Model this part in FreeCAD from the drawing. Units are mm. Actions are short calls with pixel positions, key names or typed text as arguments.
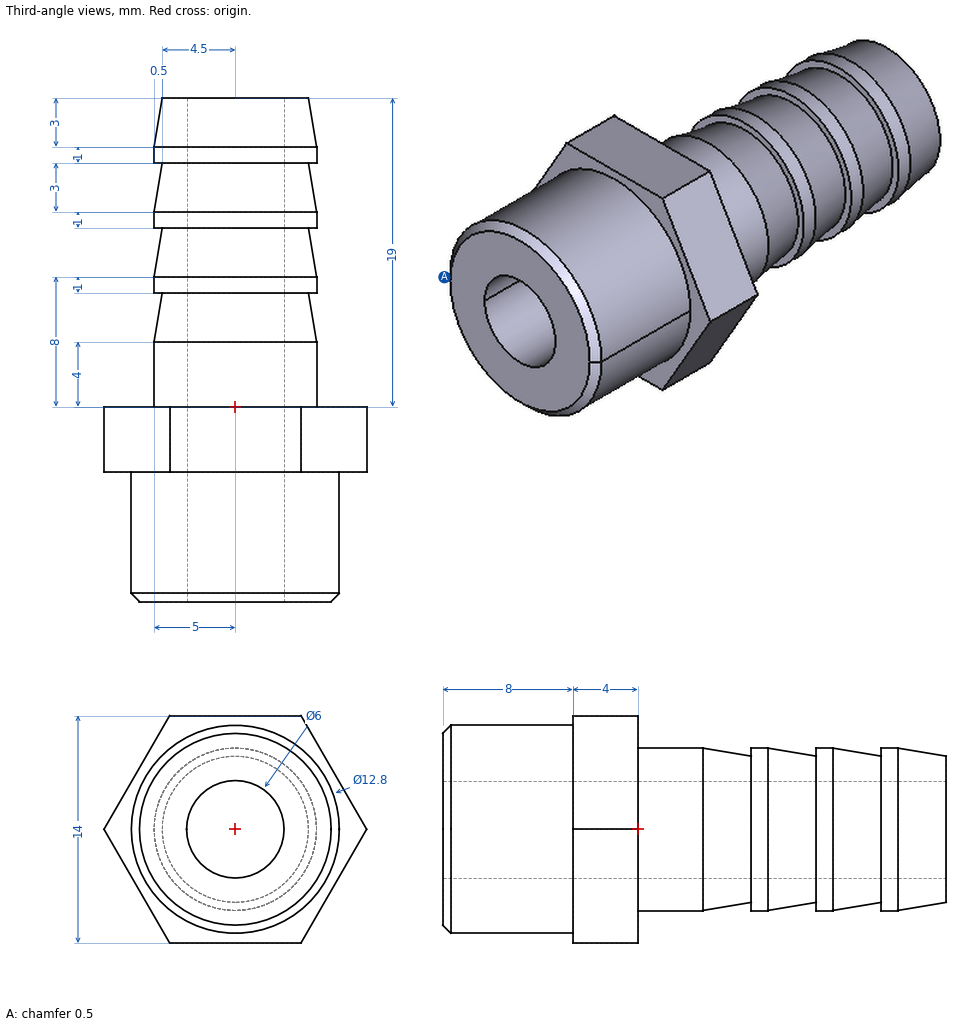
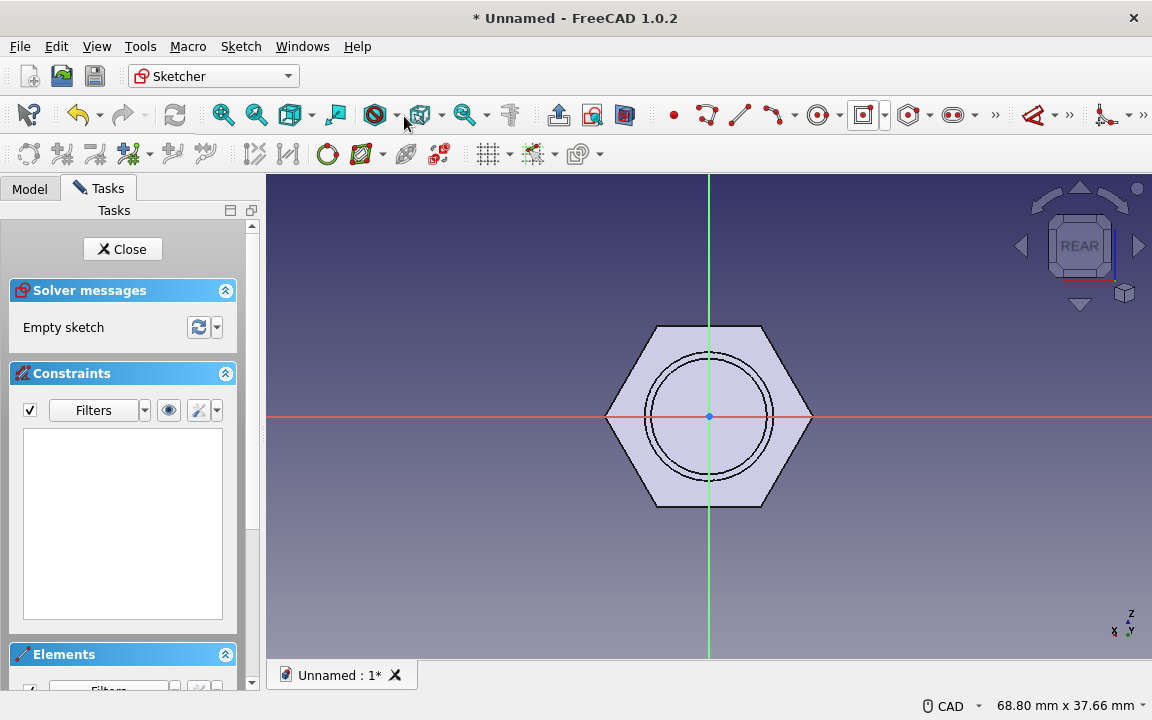
scroll(731, 417, up, 7)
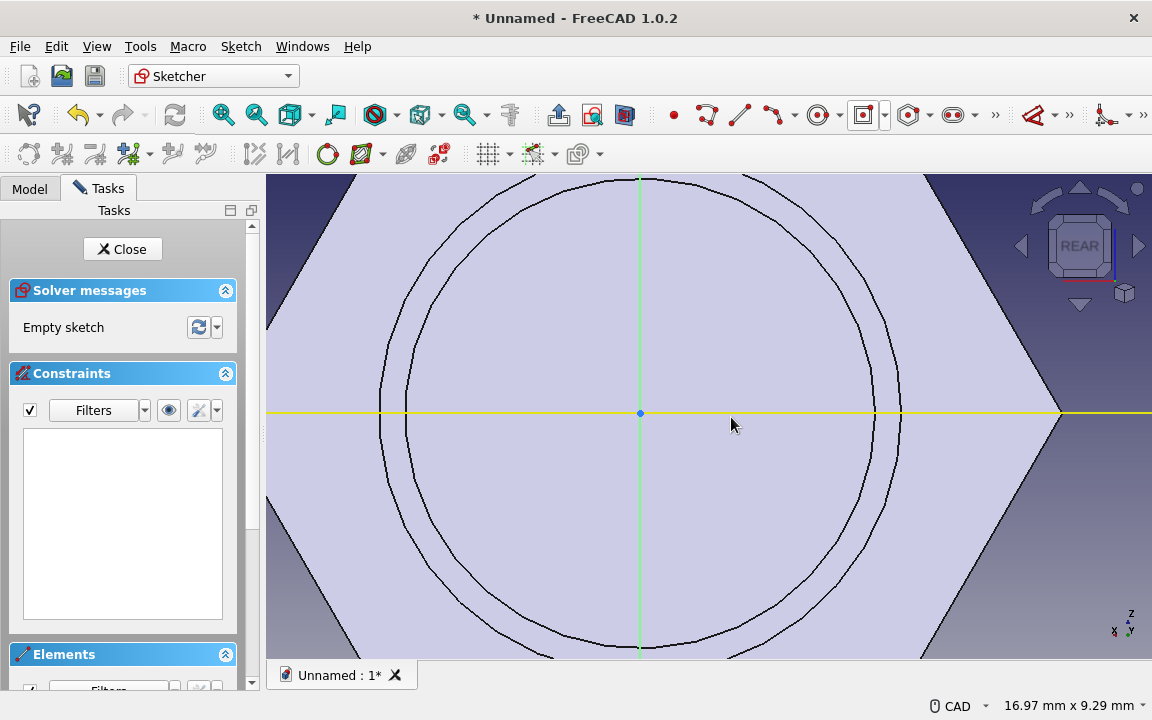
click(818, 116)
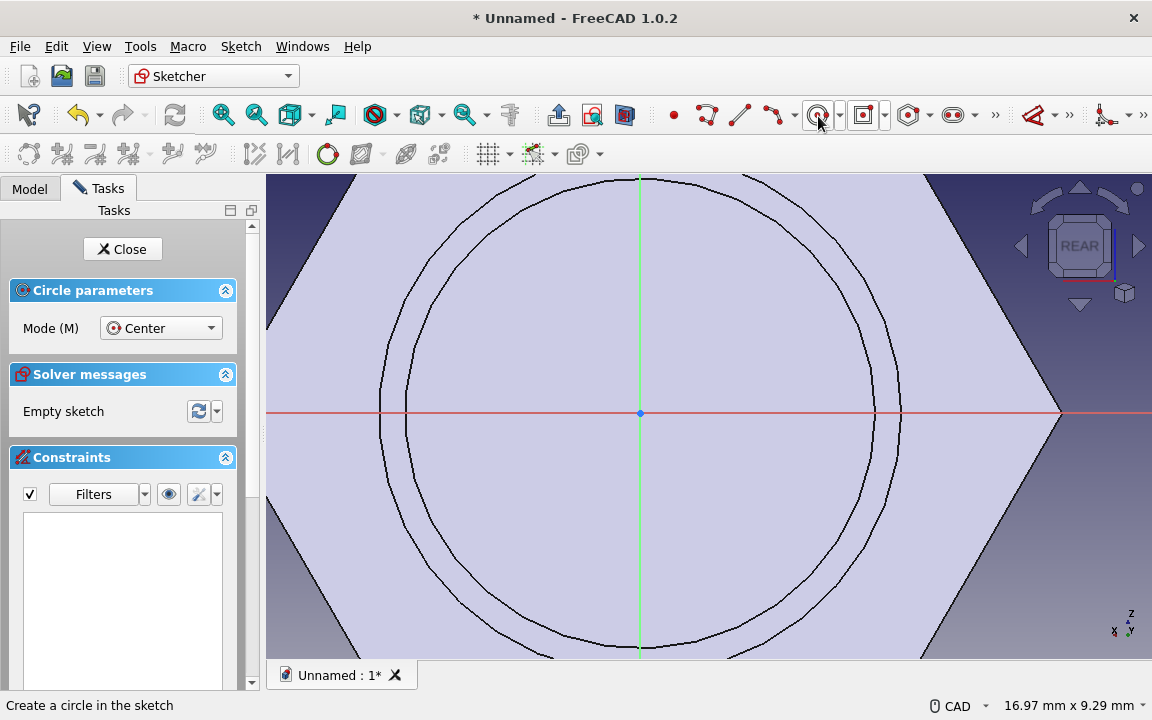
click(640, 413)
click(751, 303)
key(Escape)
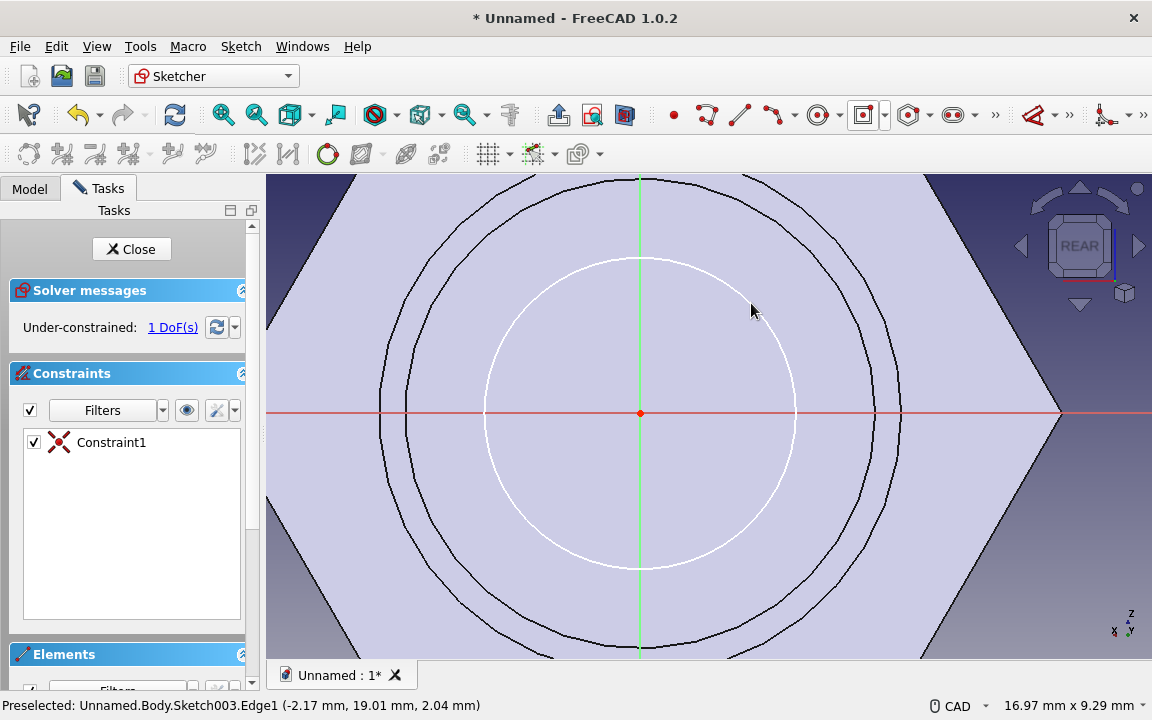
click(1032, 116)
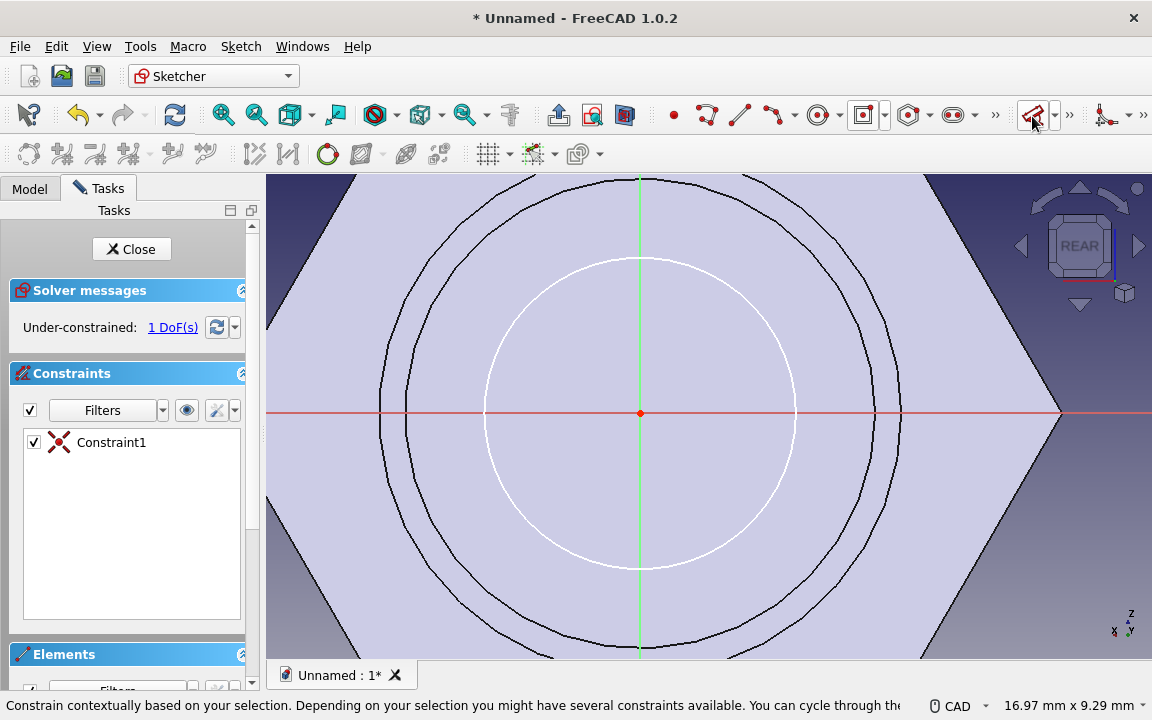
click(750, 303)
click(773, 280)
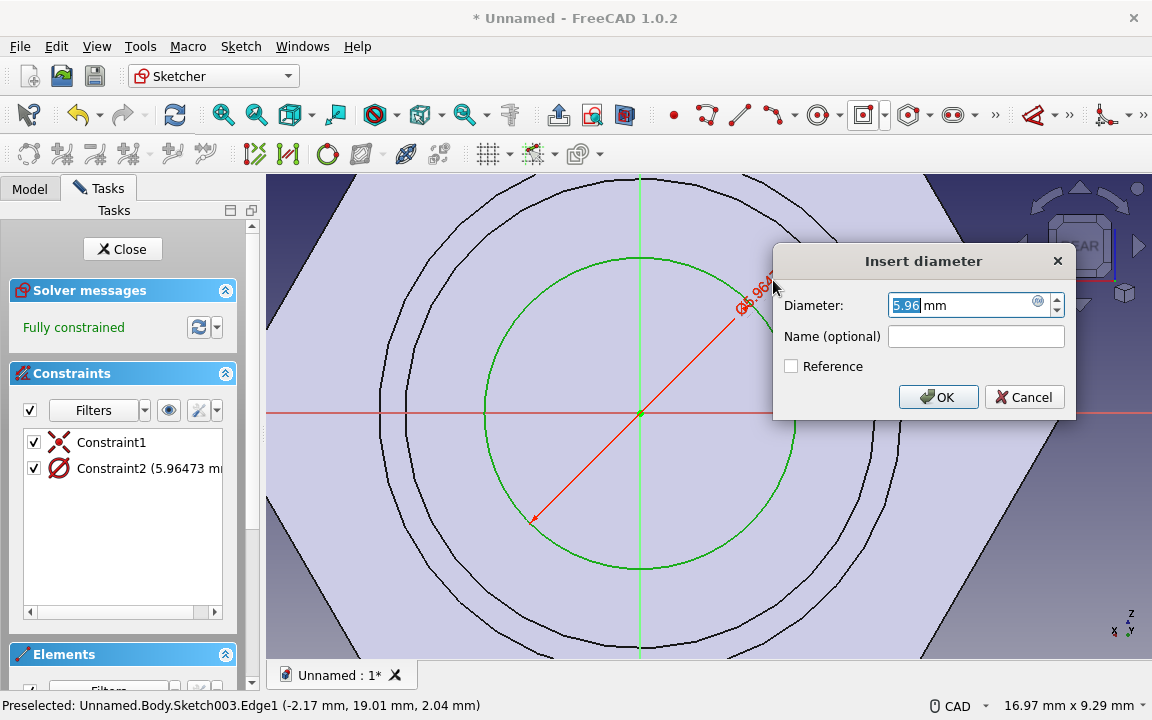
text(6)
key(Return)
key(Escape)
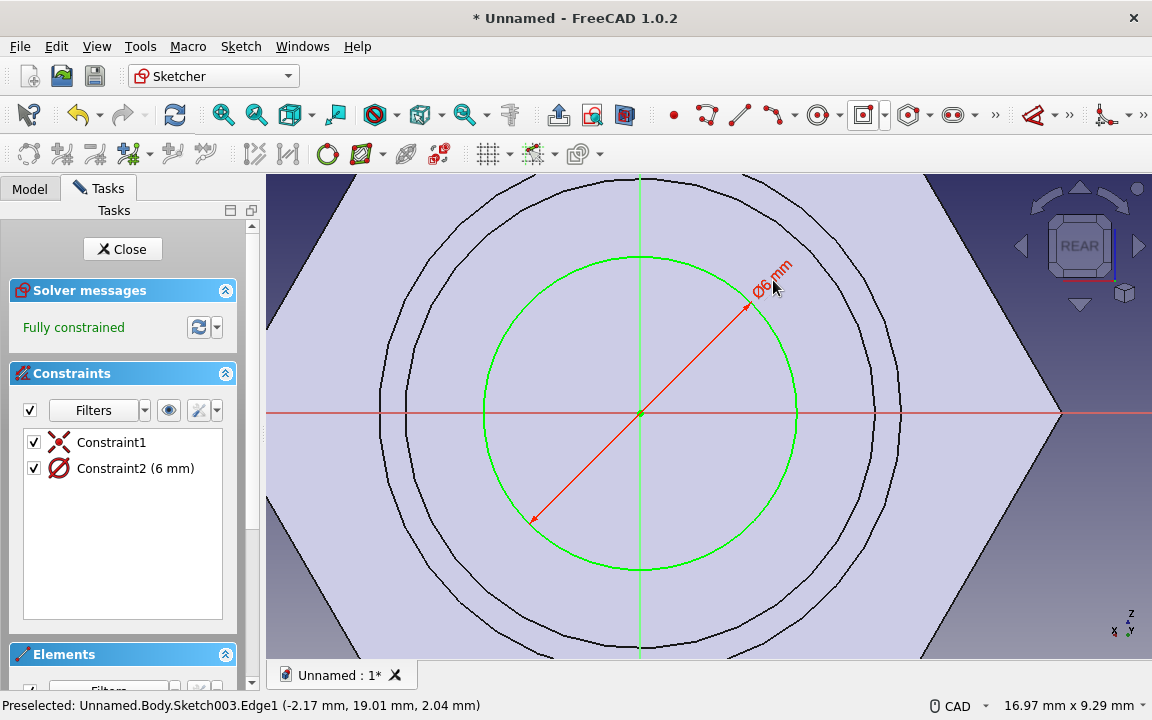
click(123, 249)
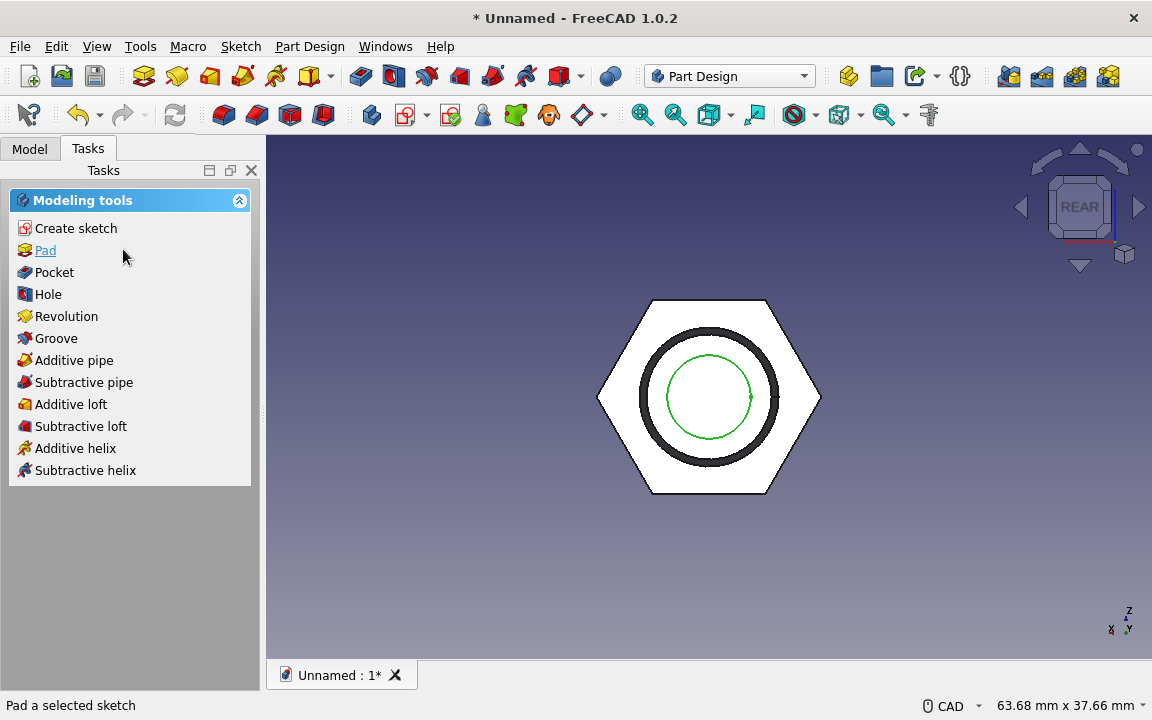
click(361, 76)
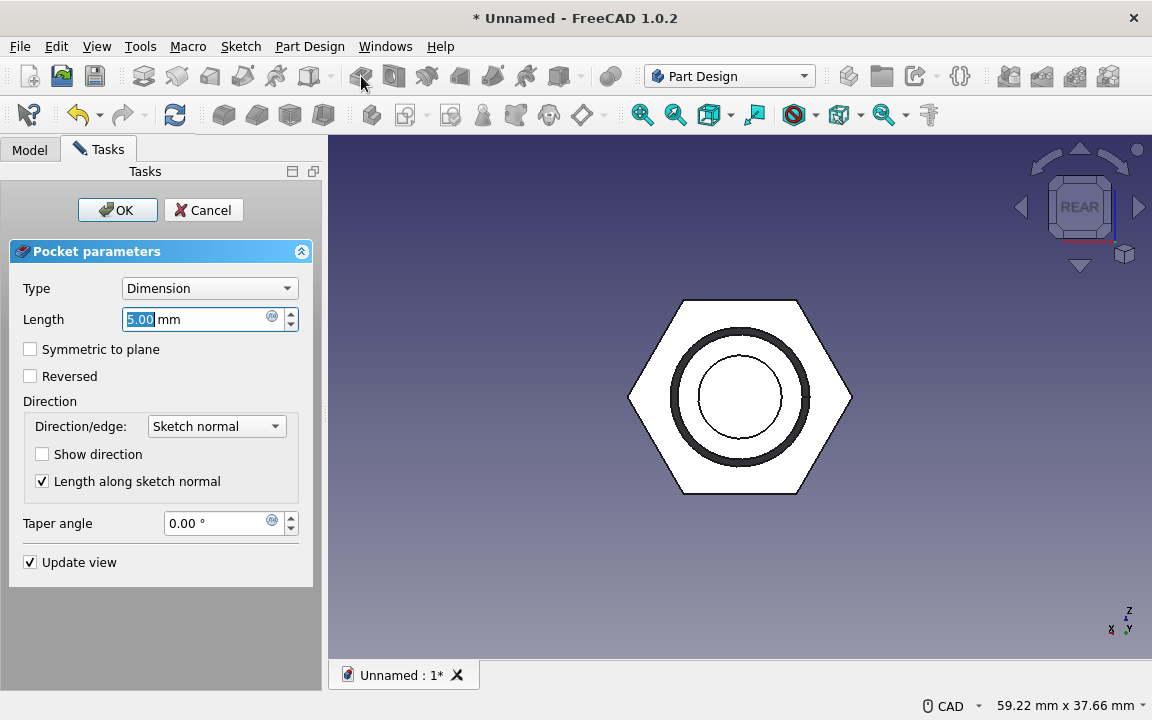
click(210, 288)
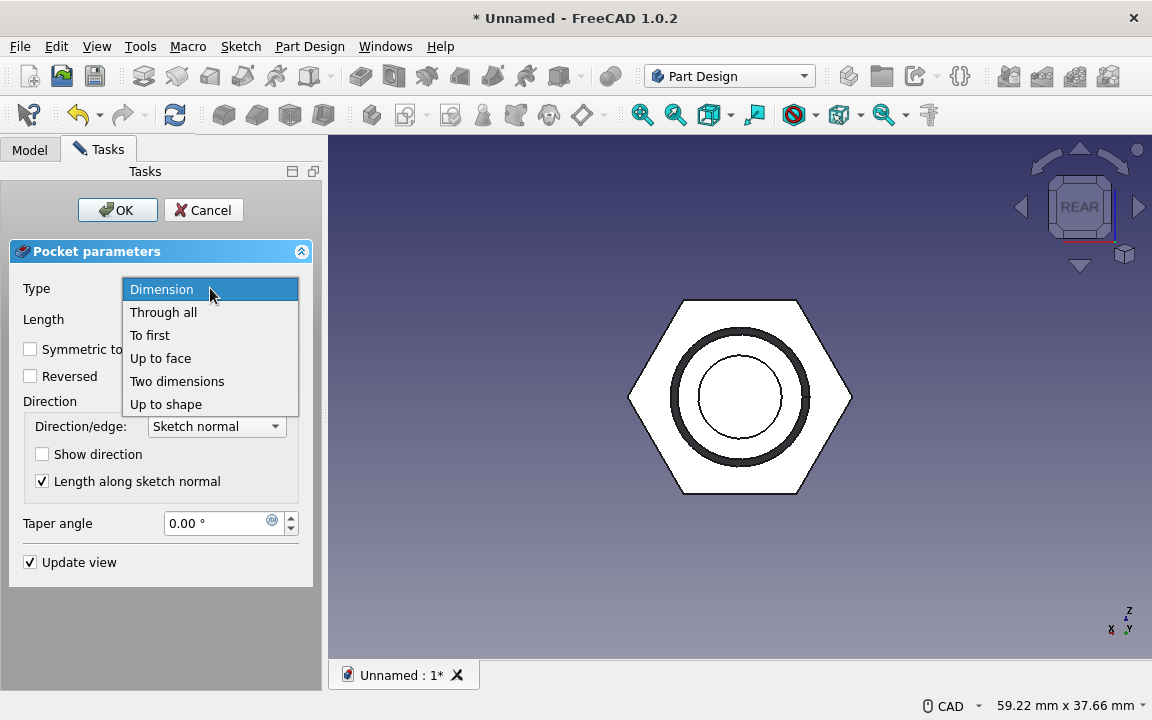
click(208, 336)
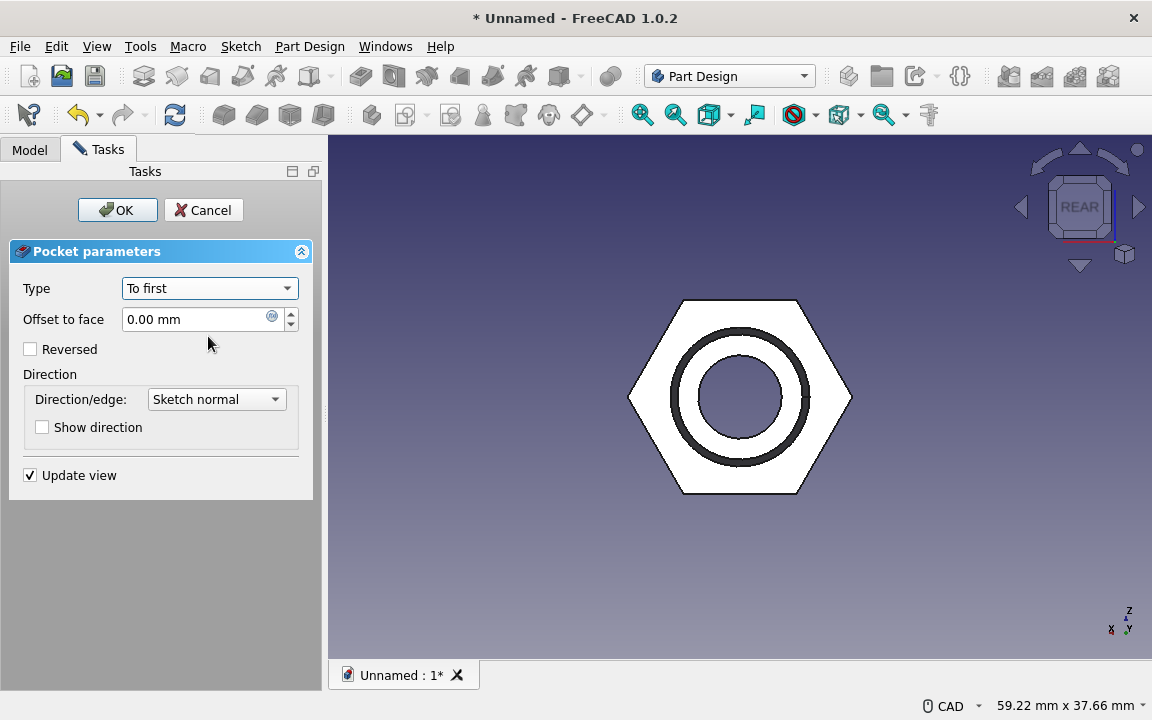
click(118, 210)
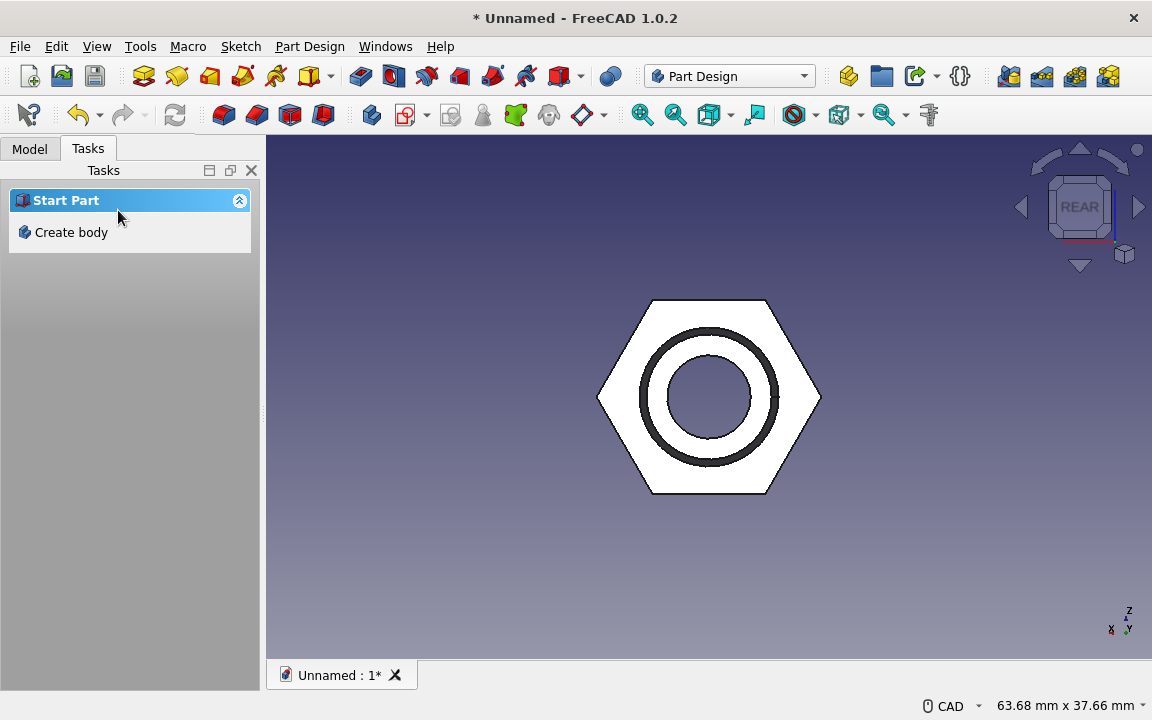
click(643, 116)